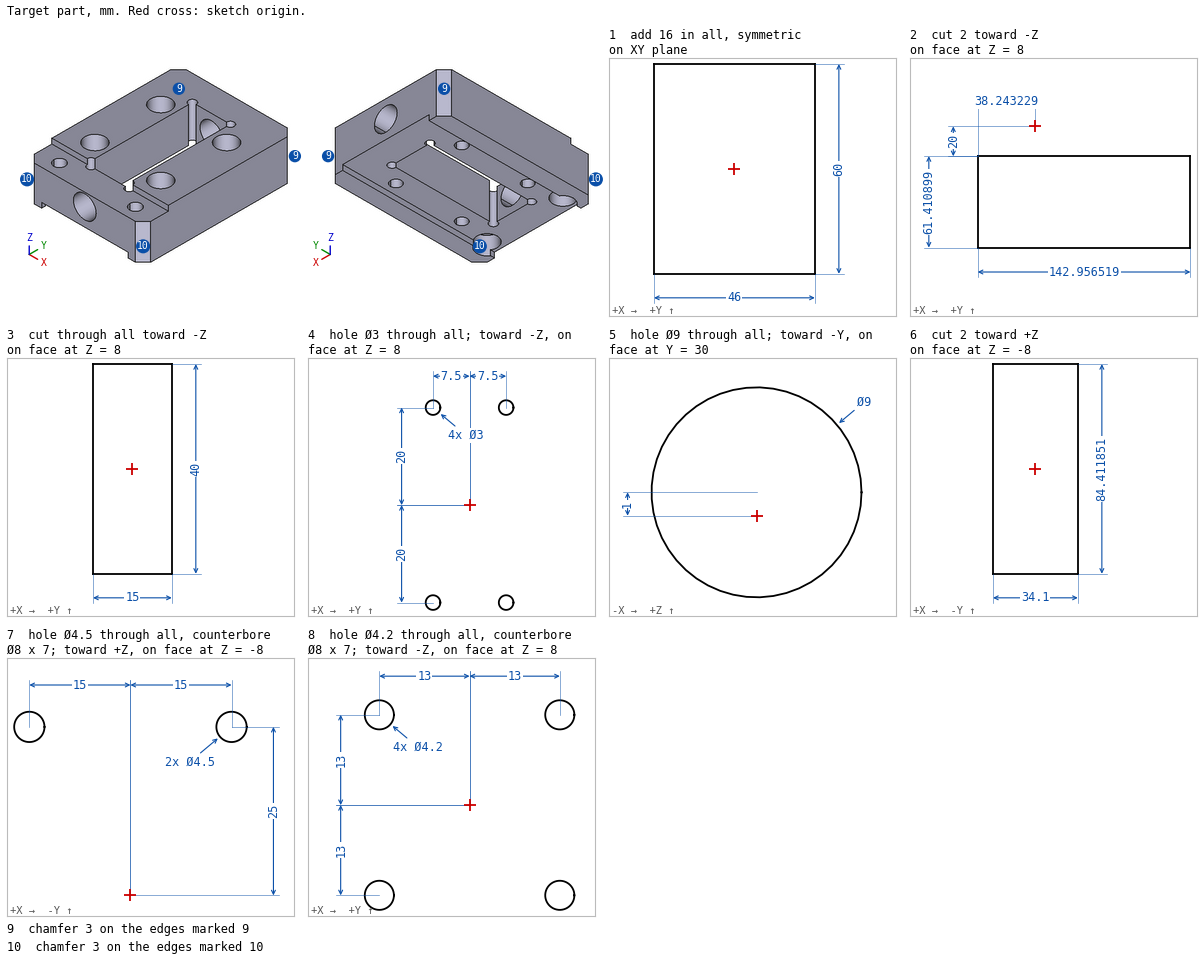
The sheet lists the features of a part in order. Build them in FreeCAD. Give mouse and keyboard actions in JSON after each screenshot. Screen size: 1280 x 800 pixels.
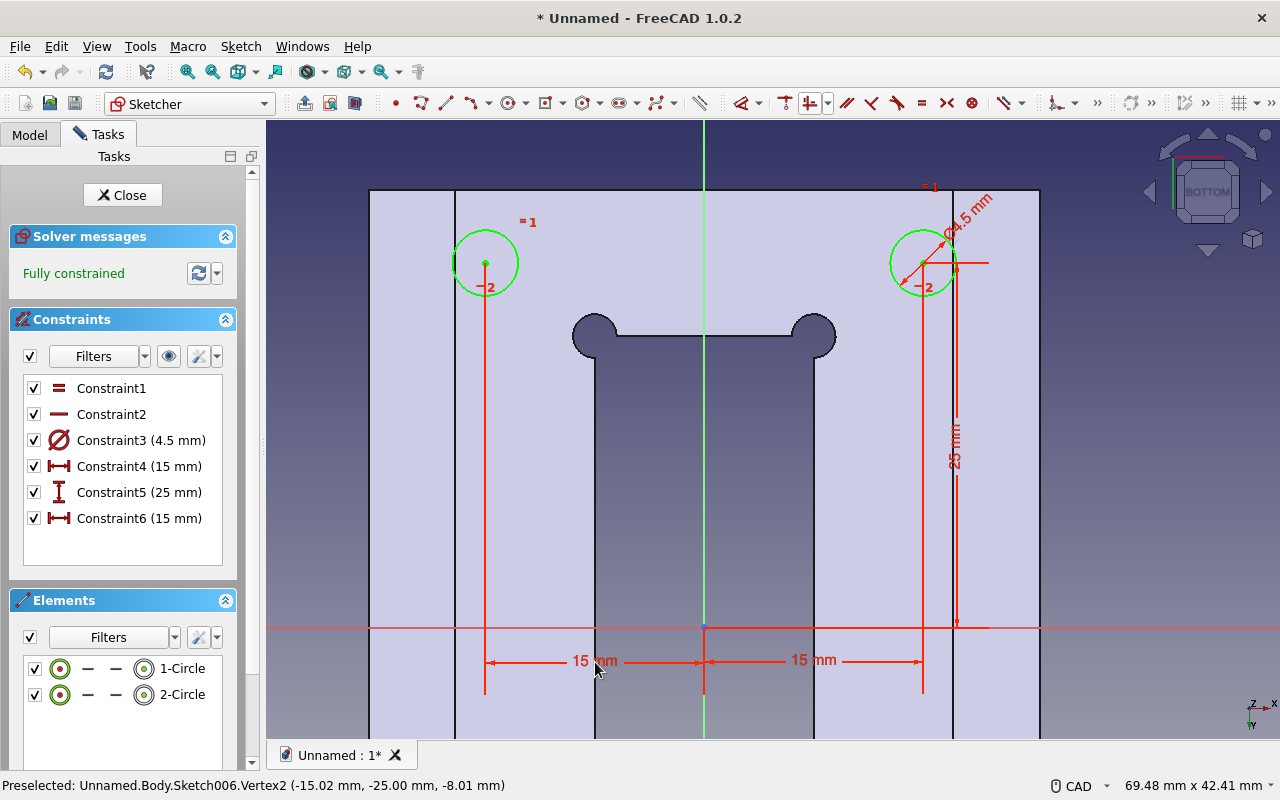
{"action": "left_click", "coordinate": [123, 195]}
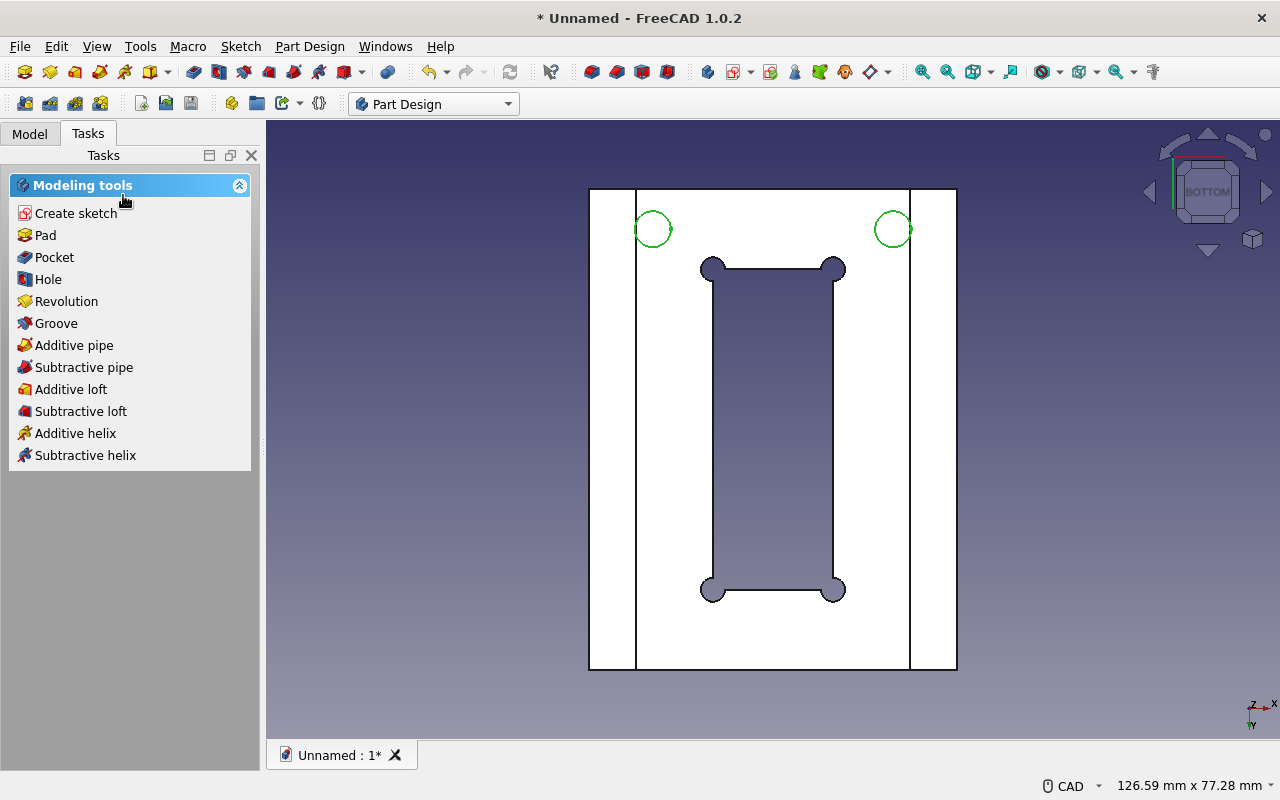
{"action": "left_click", "coordinate": [219, 72]}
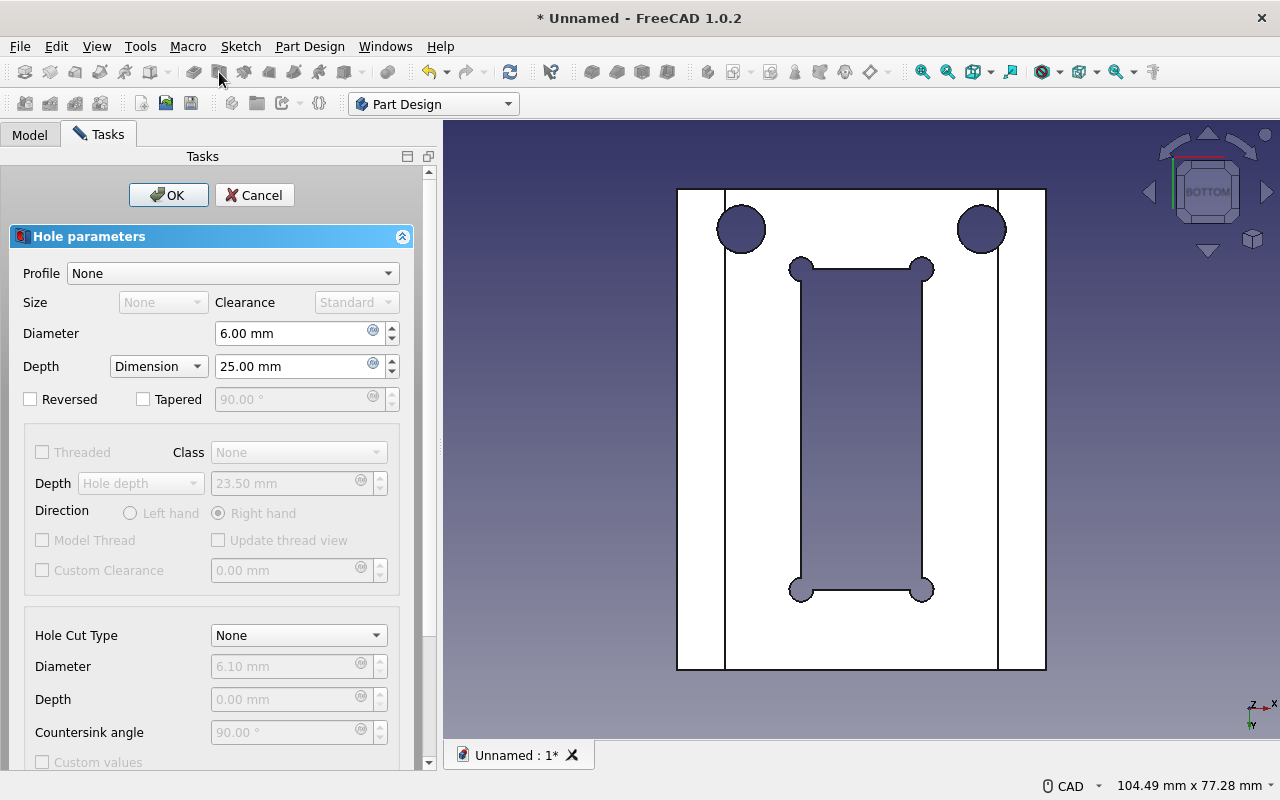
{"action": "triple_click", "coordinate": [300, 334]}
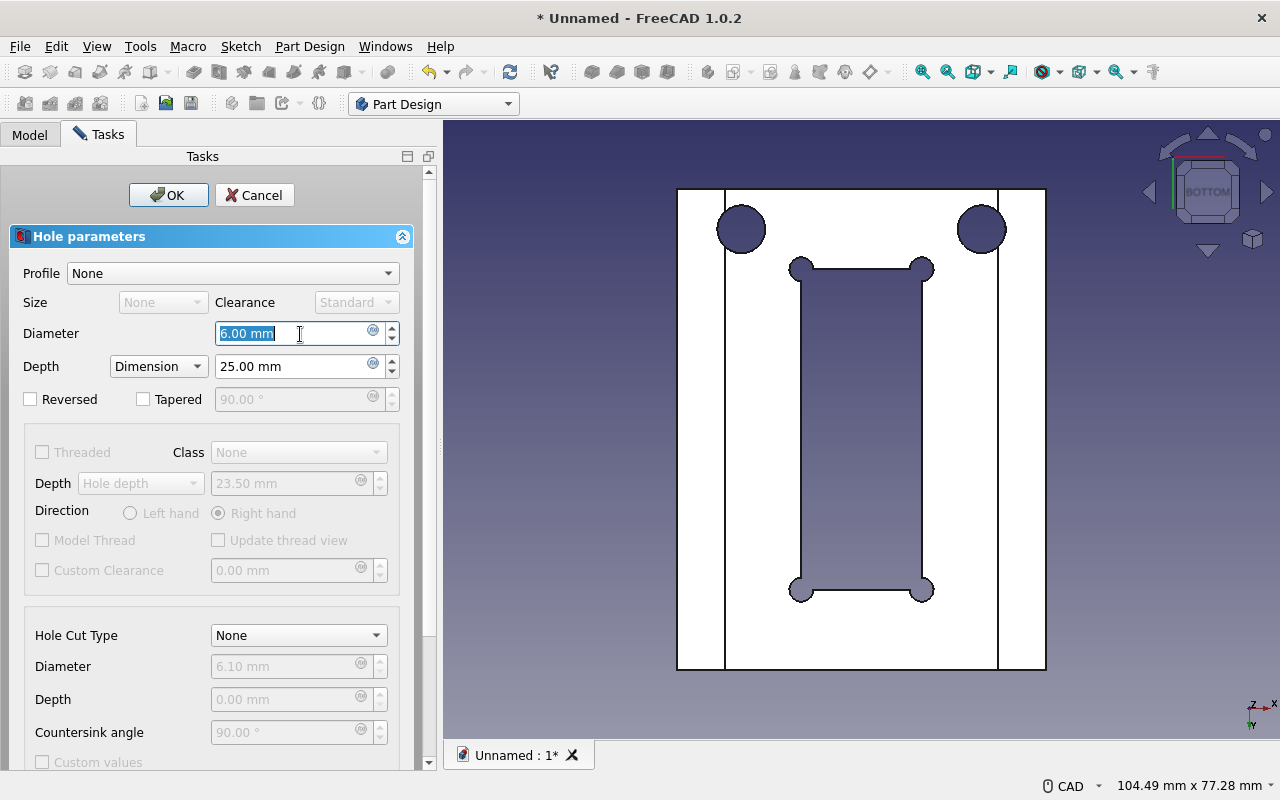
{"action": "type", "text": "4.5"}
{"action": "key", "text": "Tab"}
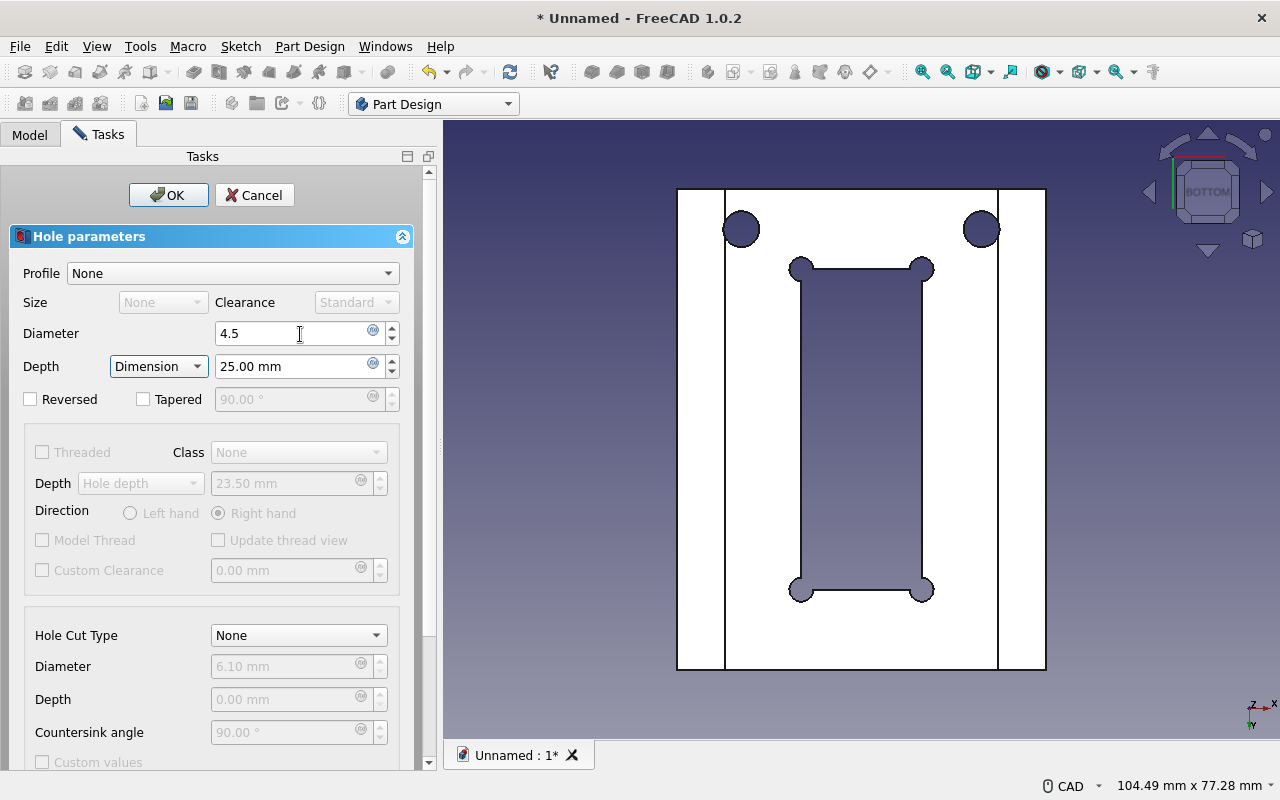
{"action": "left_click", "coordinate": [160, 366]}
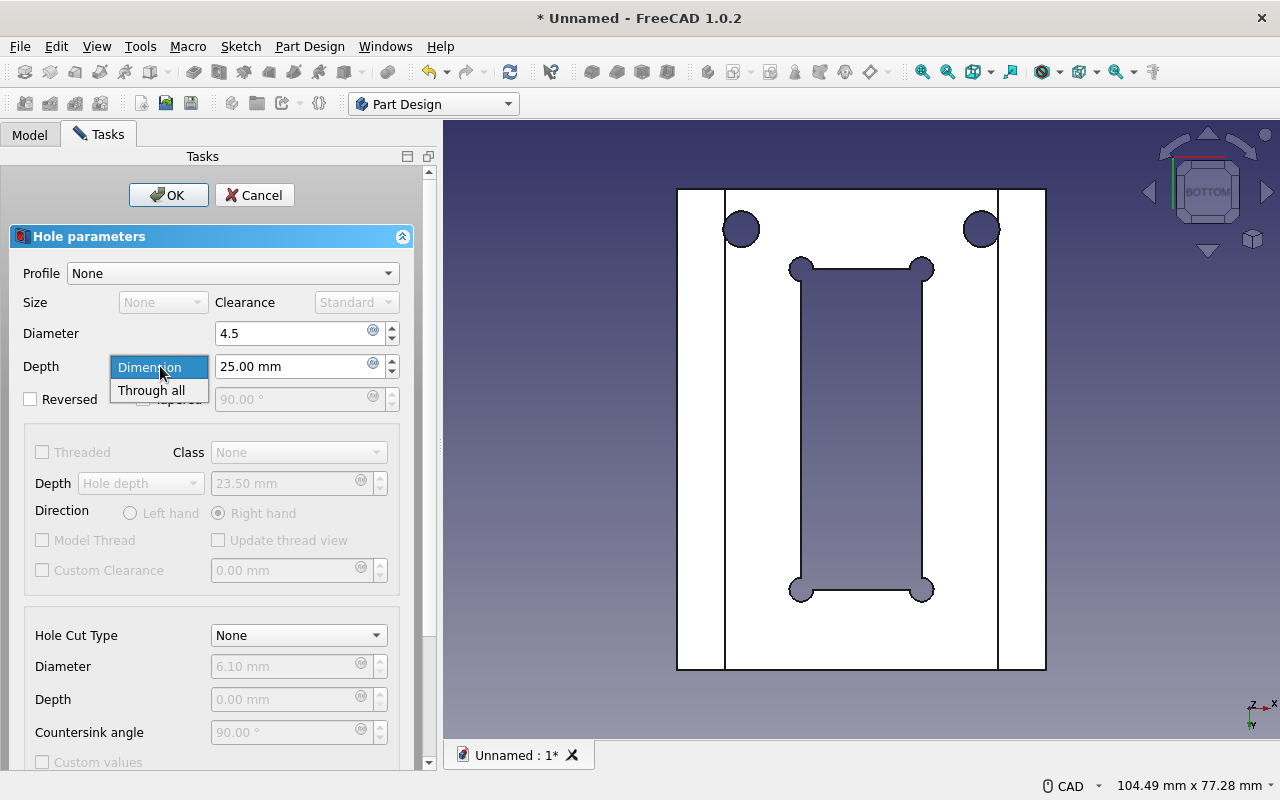
{"action": "left_click", "coordinate": [158, 390]}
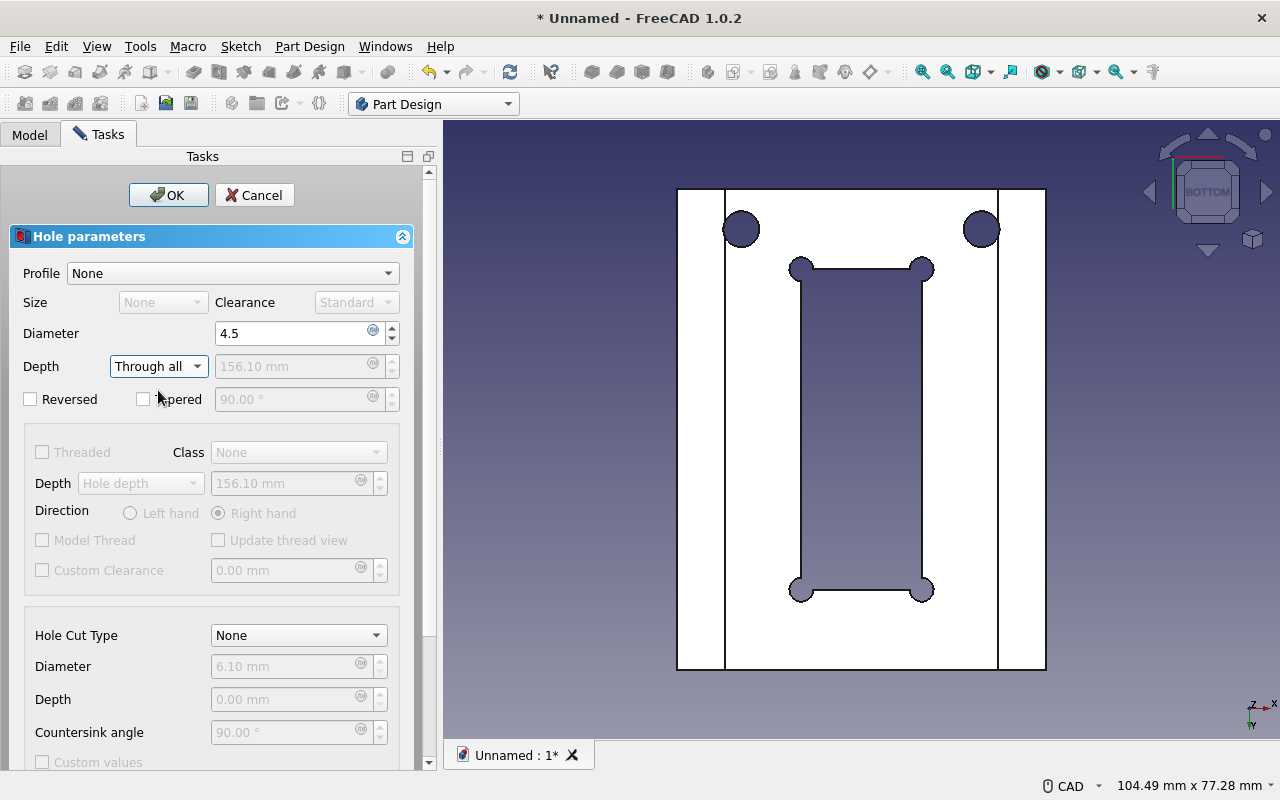
{"action": "left_click", "coordinate": [300, 636]}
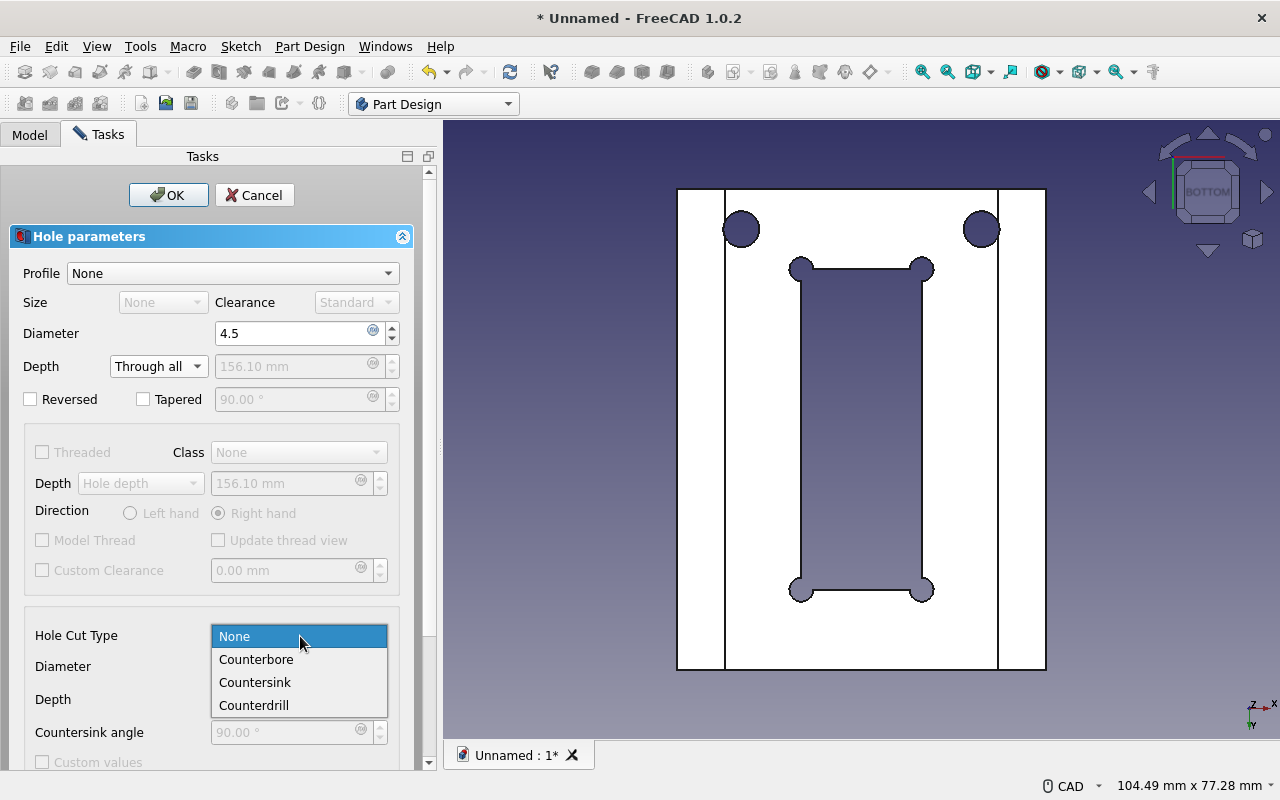
{"action": "left_click", "coordinate": [298, 660]}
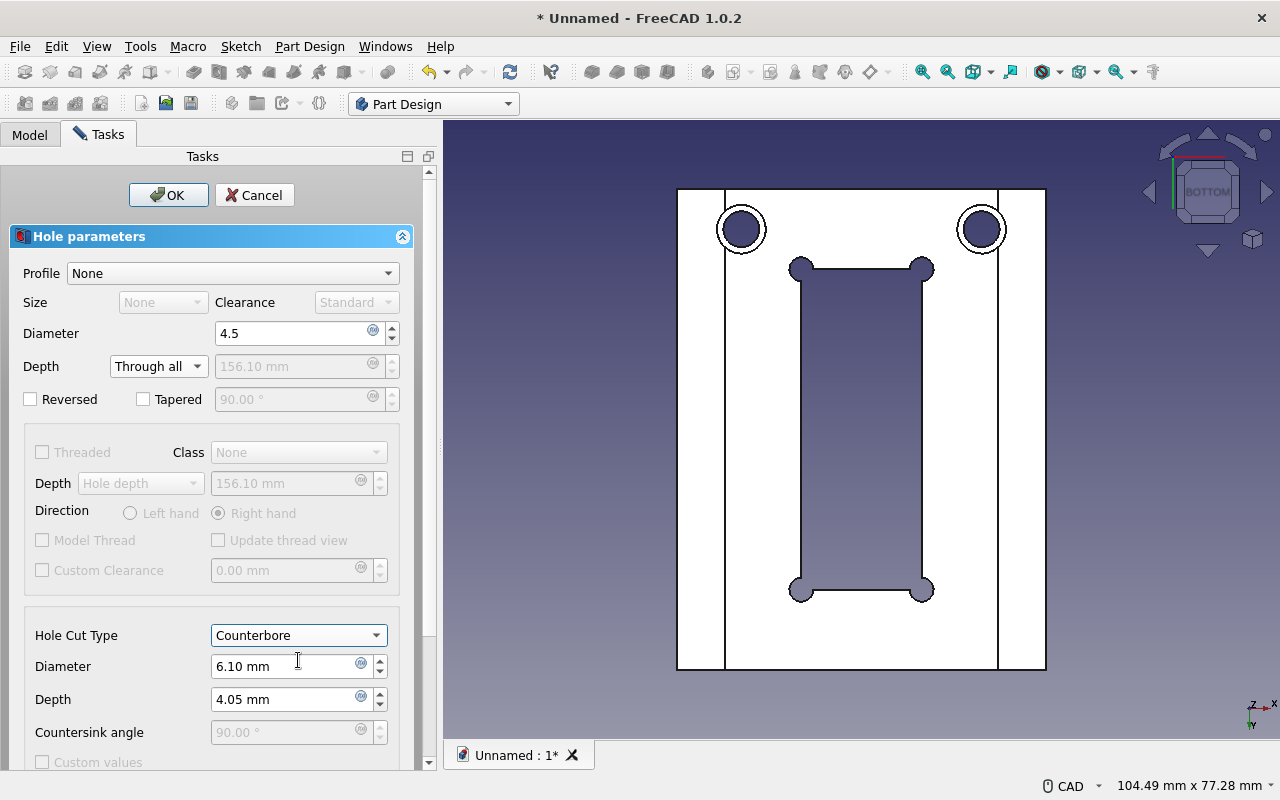
{"action": "triple_click", "coordinate": [292, 666]}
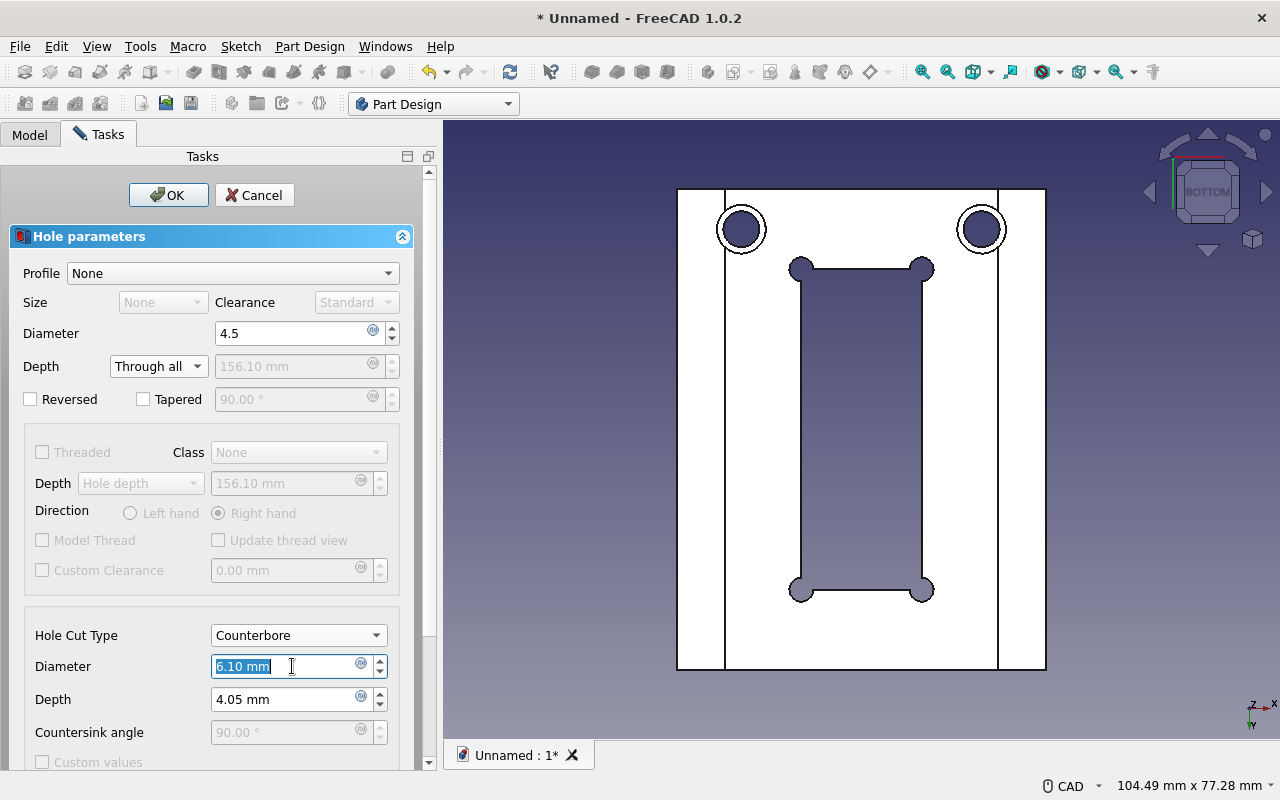
{"action": "type", "text": "8"}
{"action": "key", "text": "Tab"}